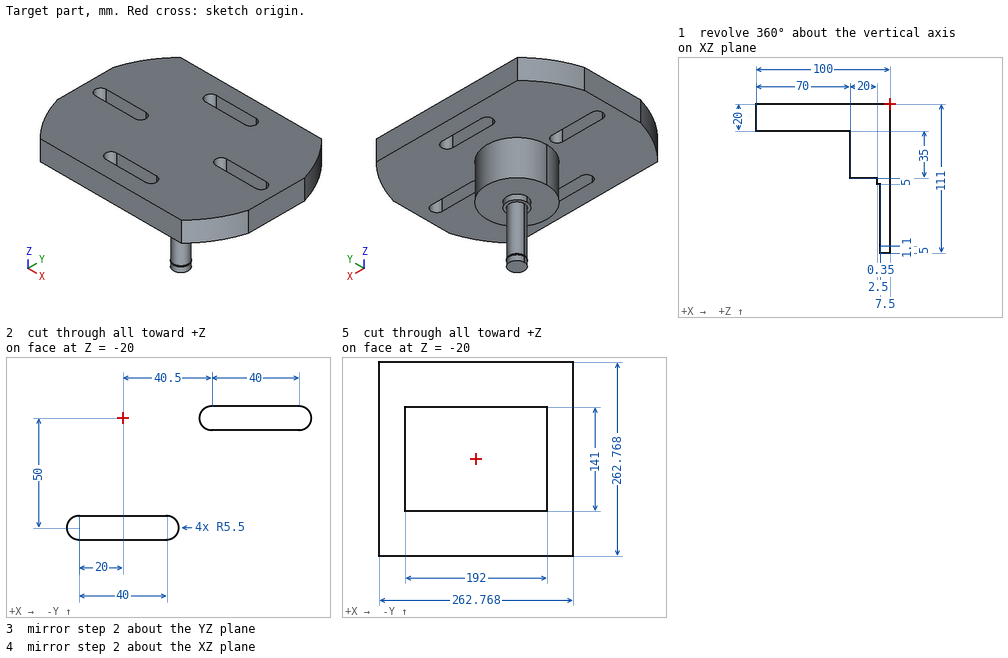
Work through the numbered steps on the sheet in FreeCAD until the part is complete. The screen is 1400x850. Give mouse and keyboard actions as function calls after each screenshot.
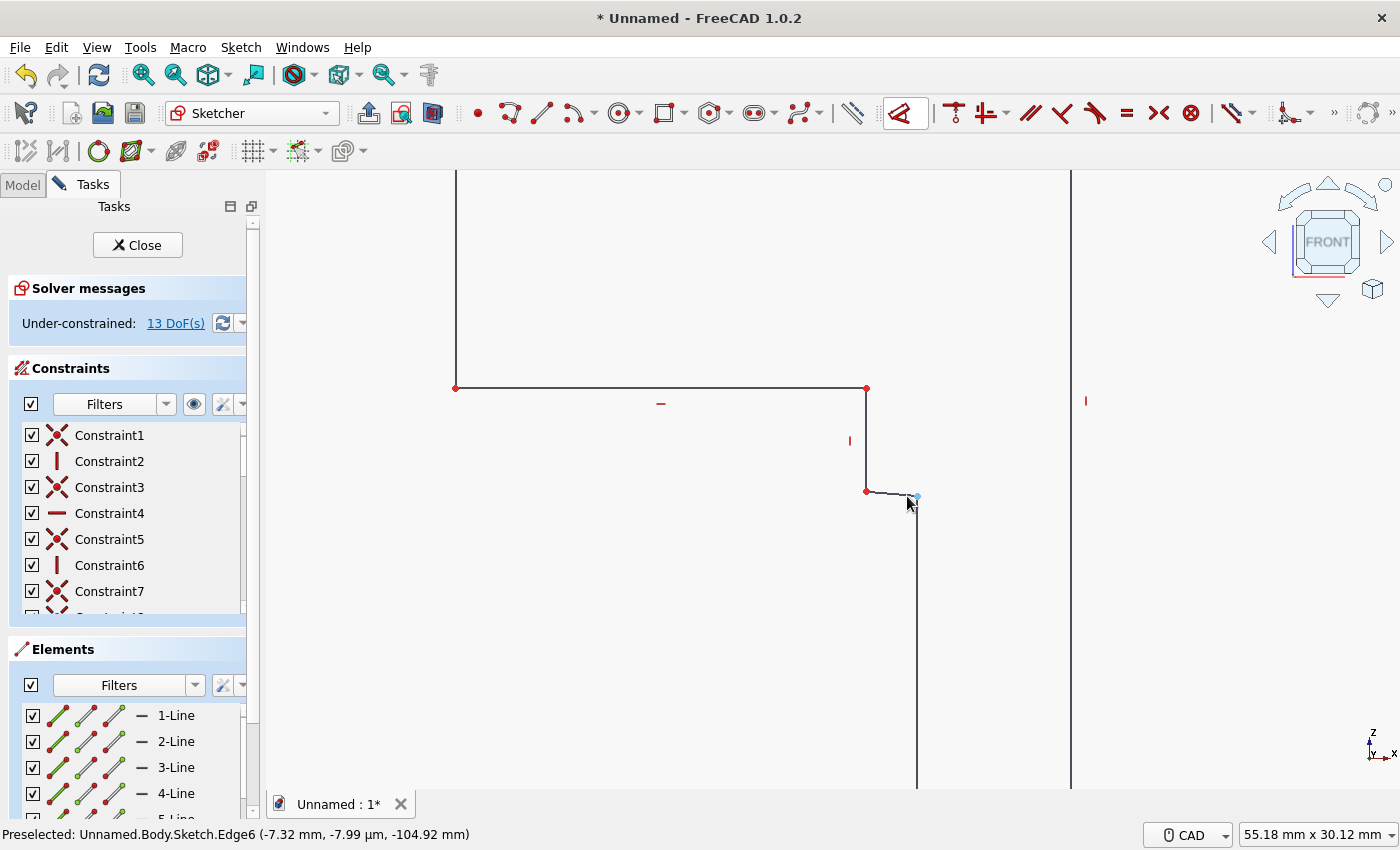
click(902, 495)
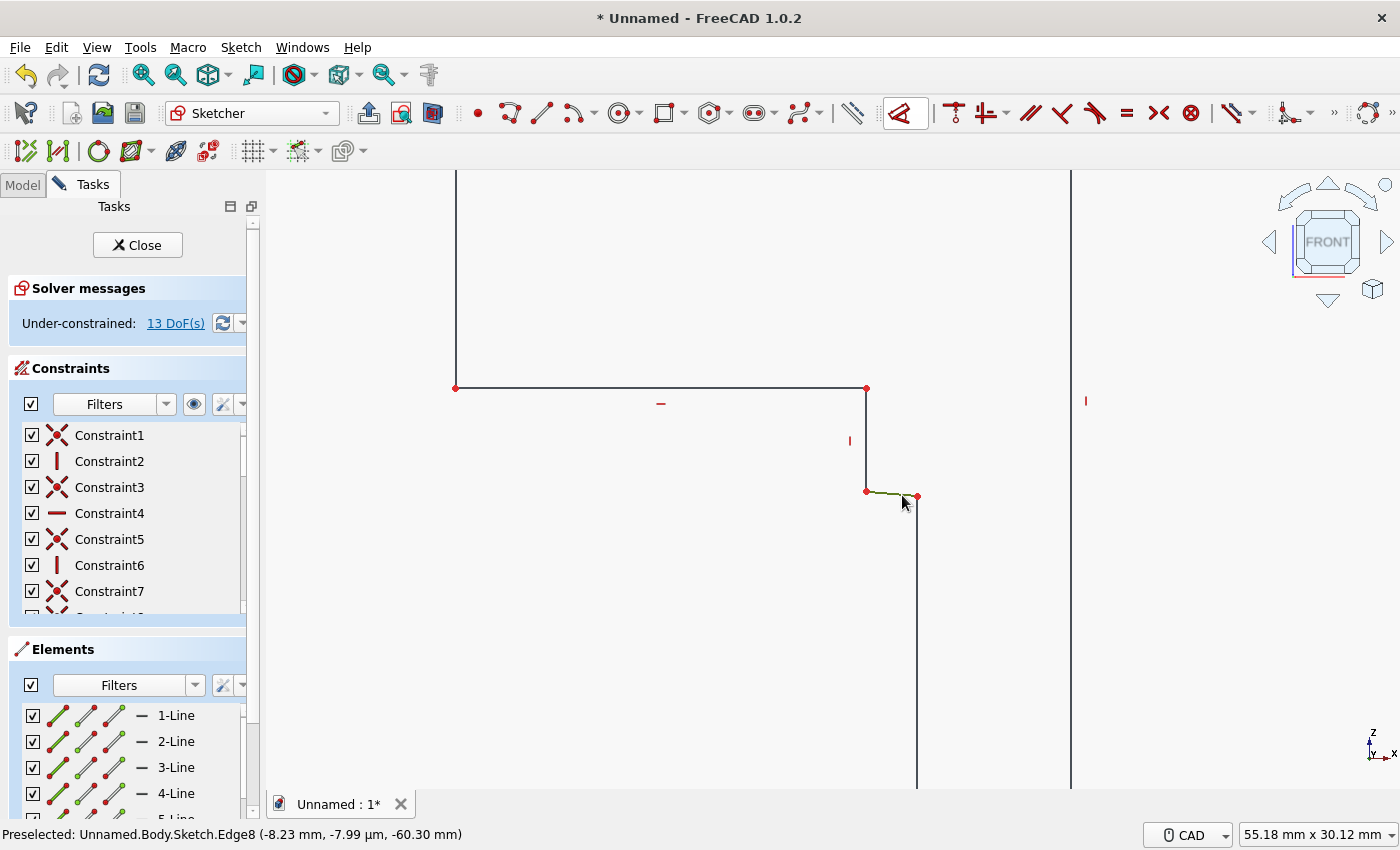
click(1008, 114)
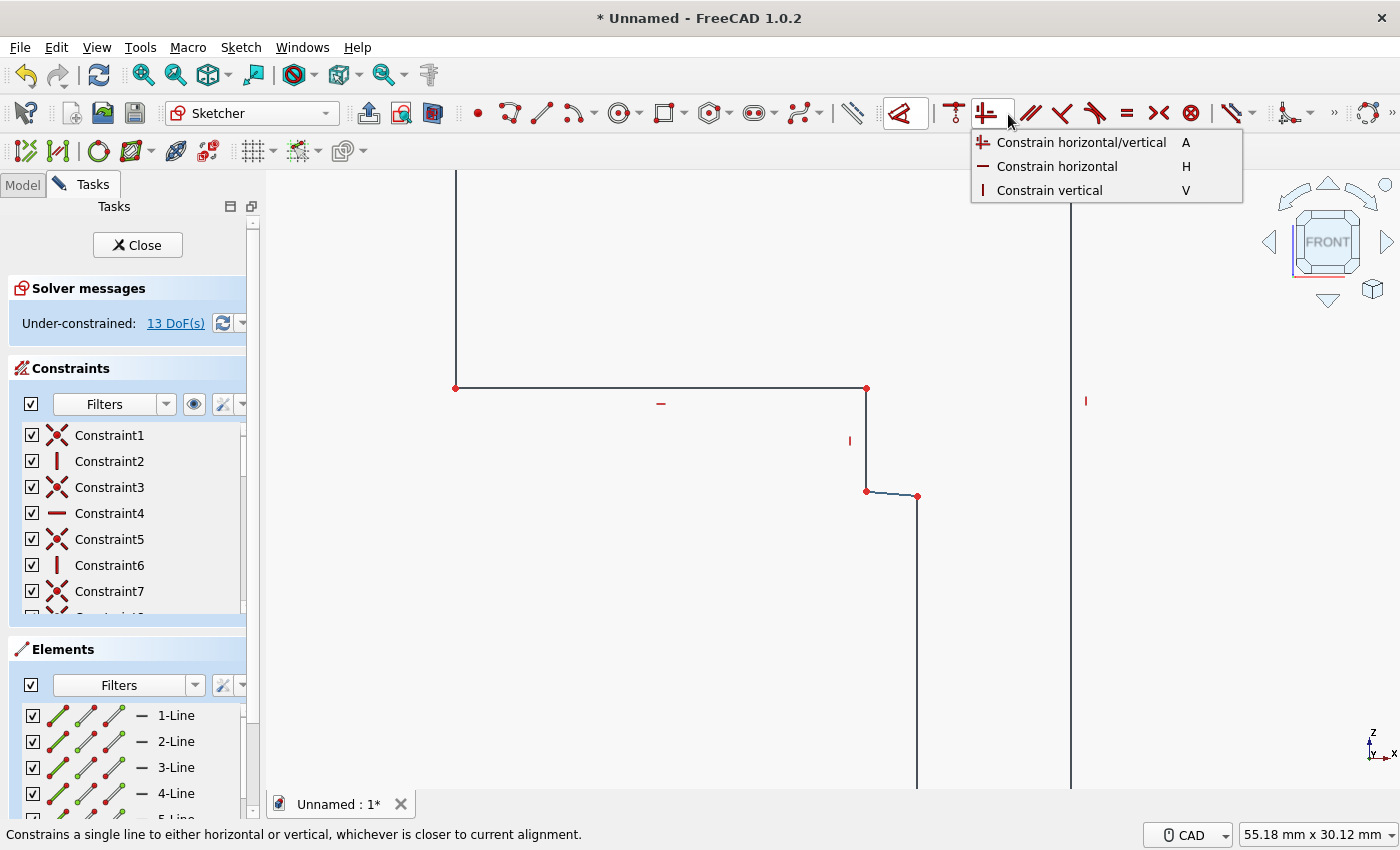
click(1107, 166)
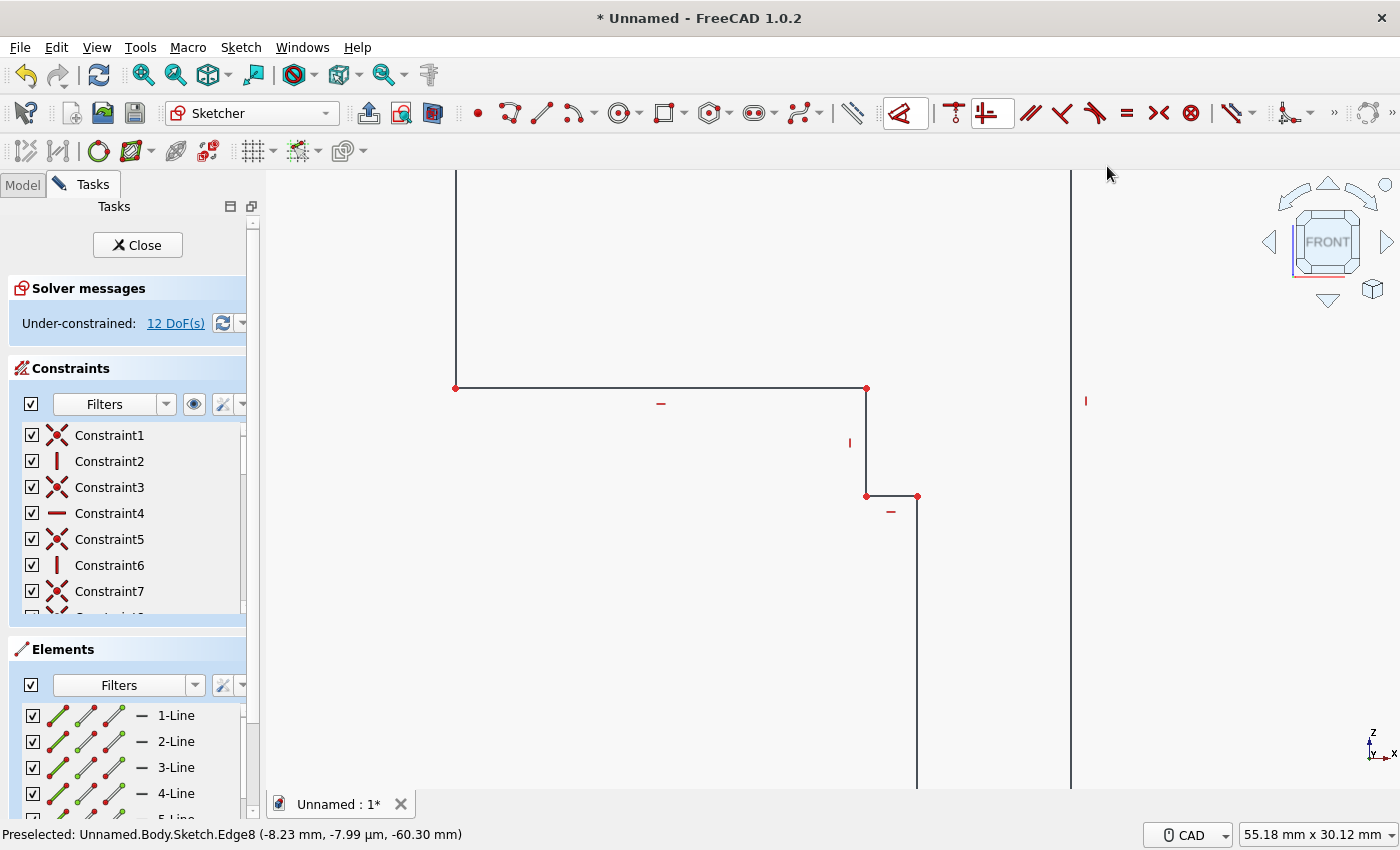
click(900, 114)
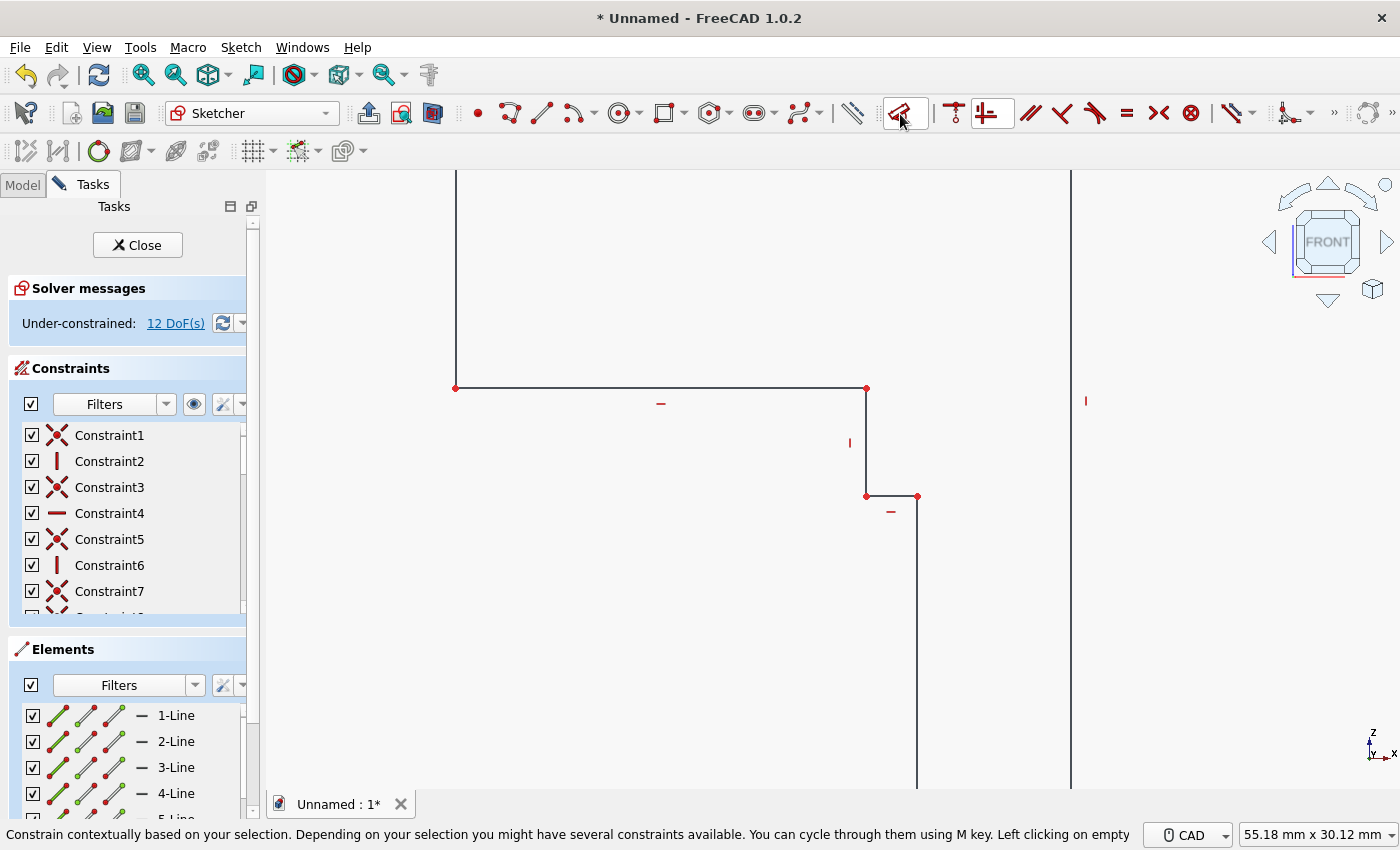
scroll(907, 496, down, 9)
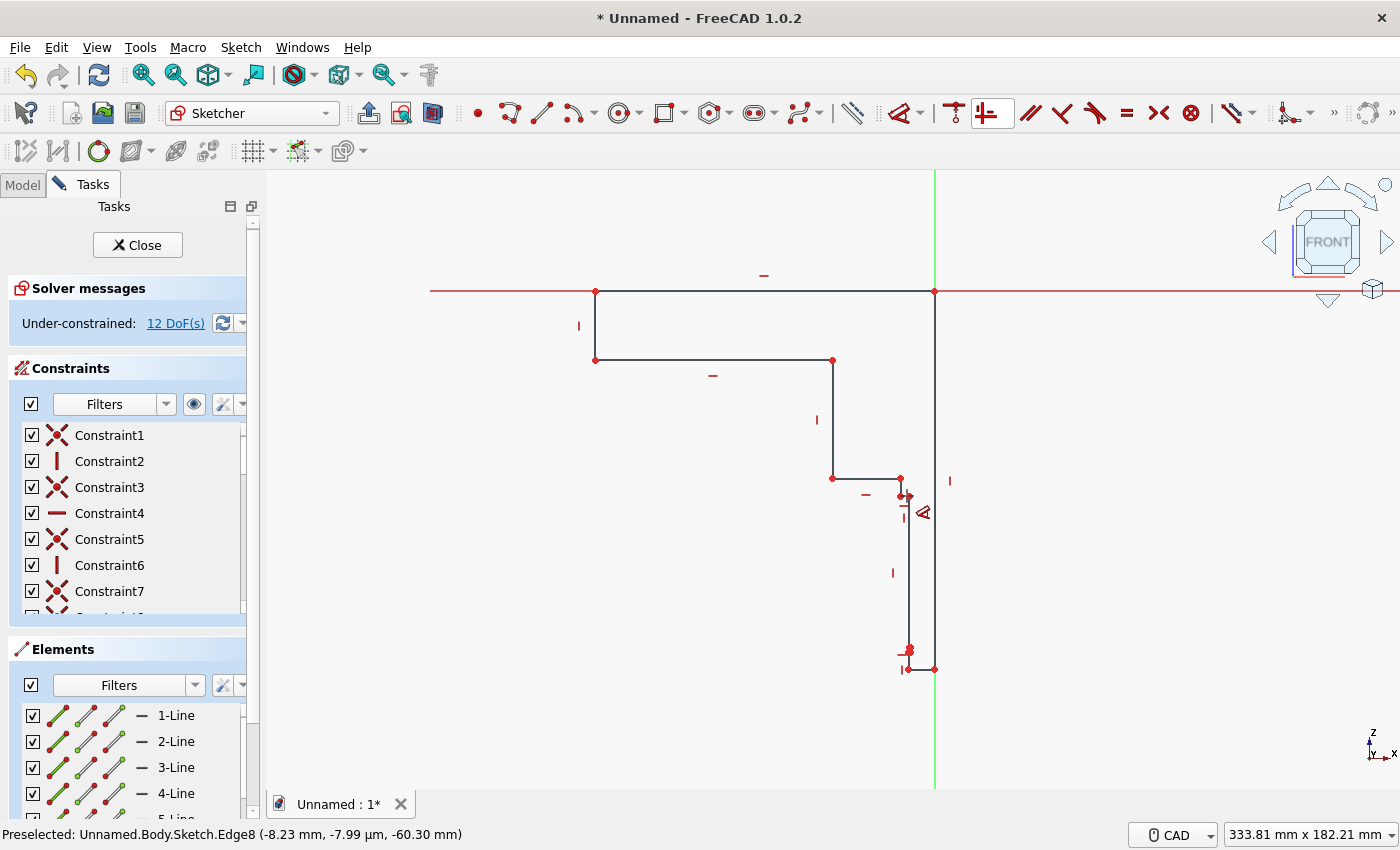
scroll(909, 665, up, 5)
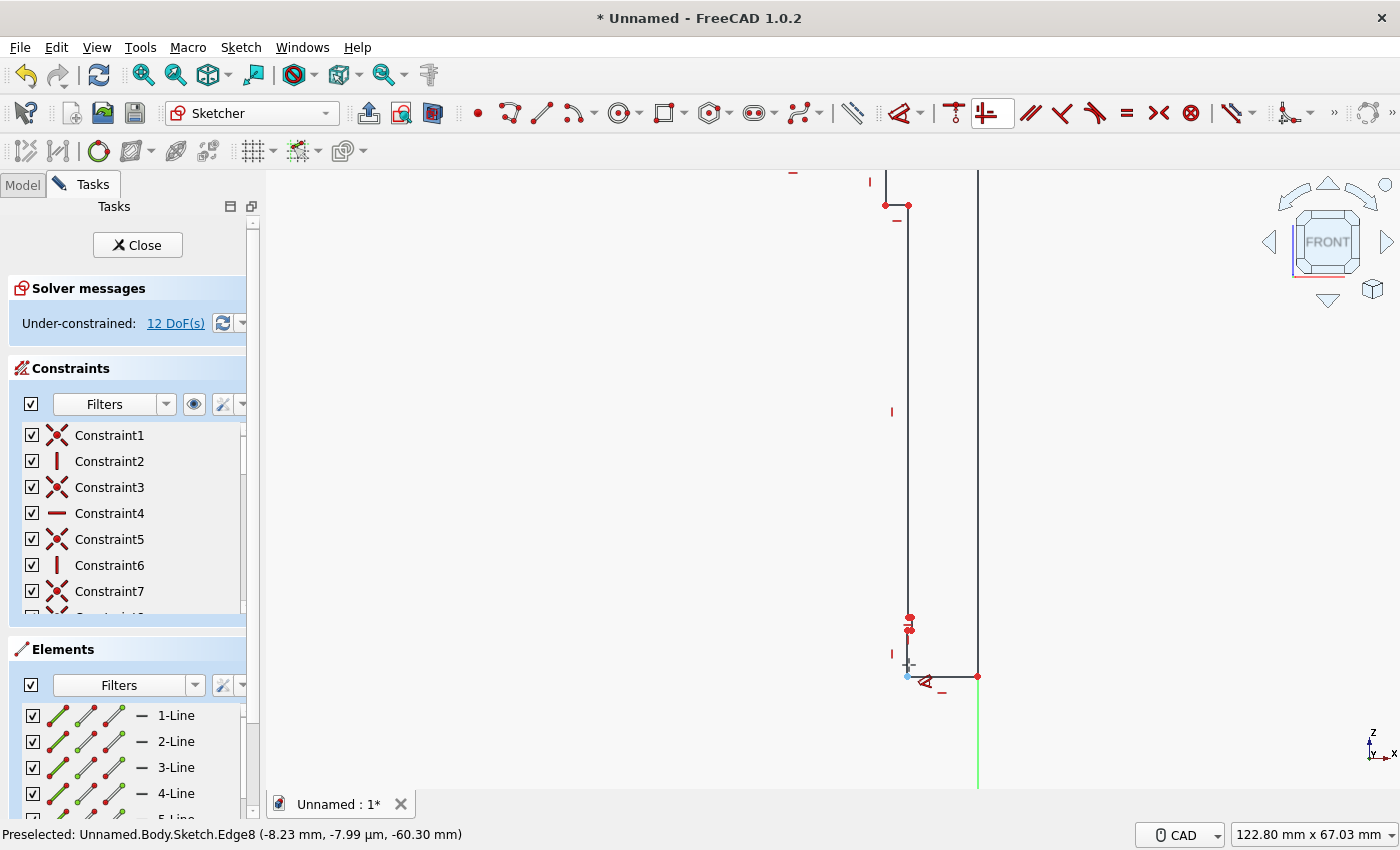
click(907, 663)
click(941, 654)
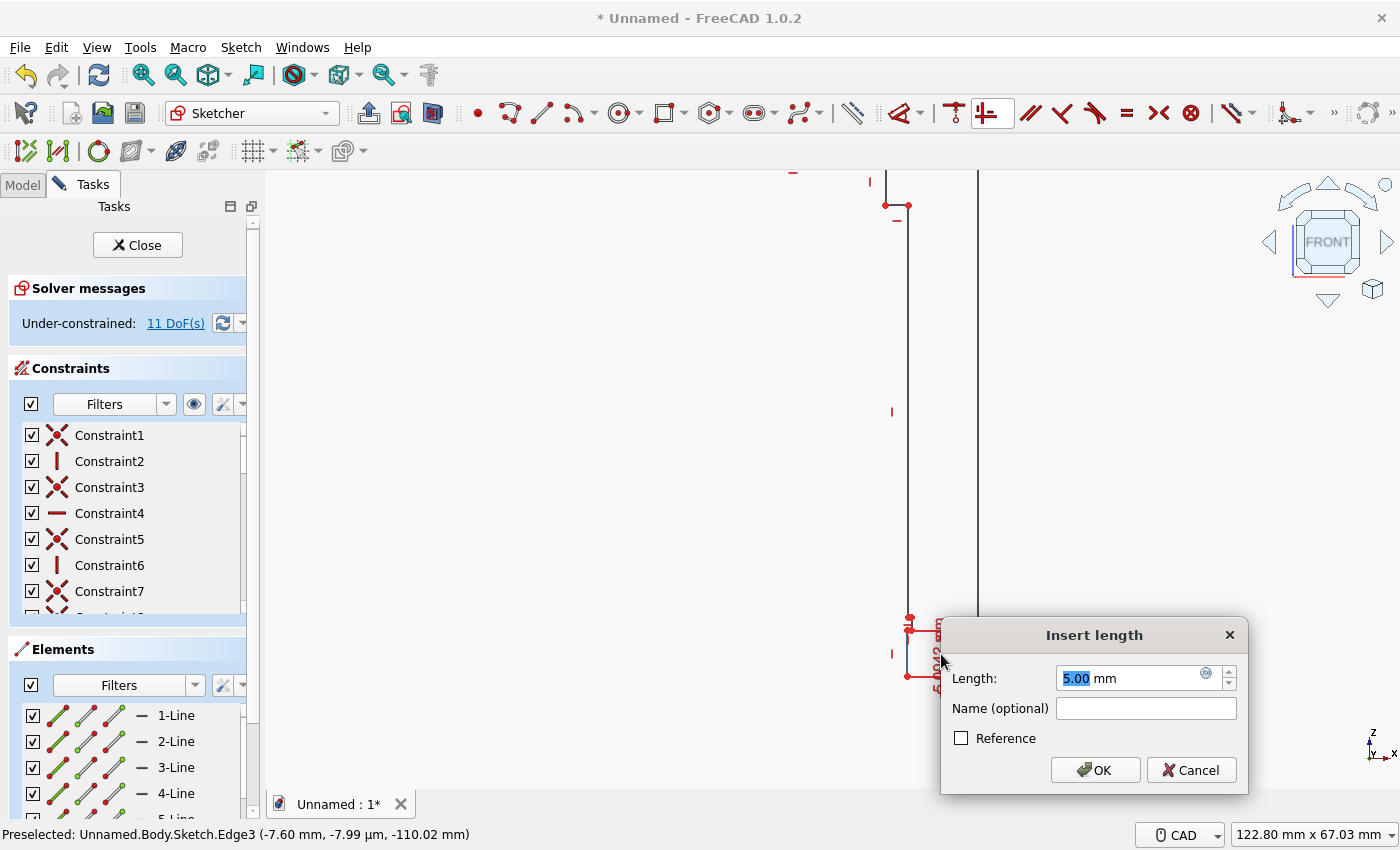
text(5)
key(Return)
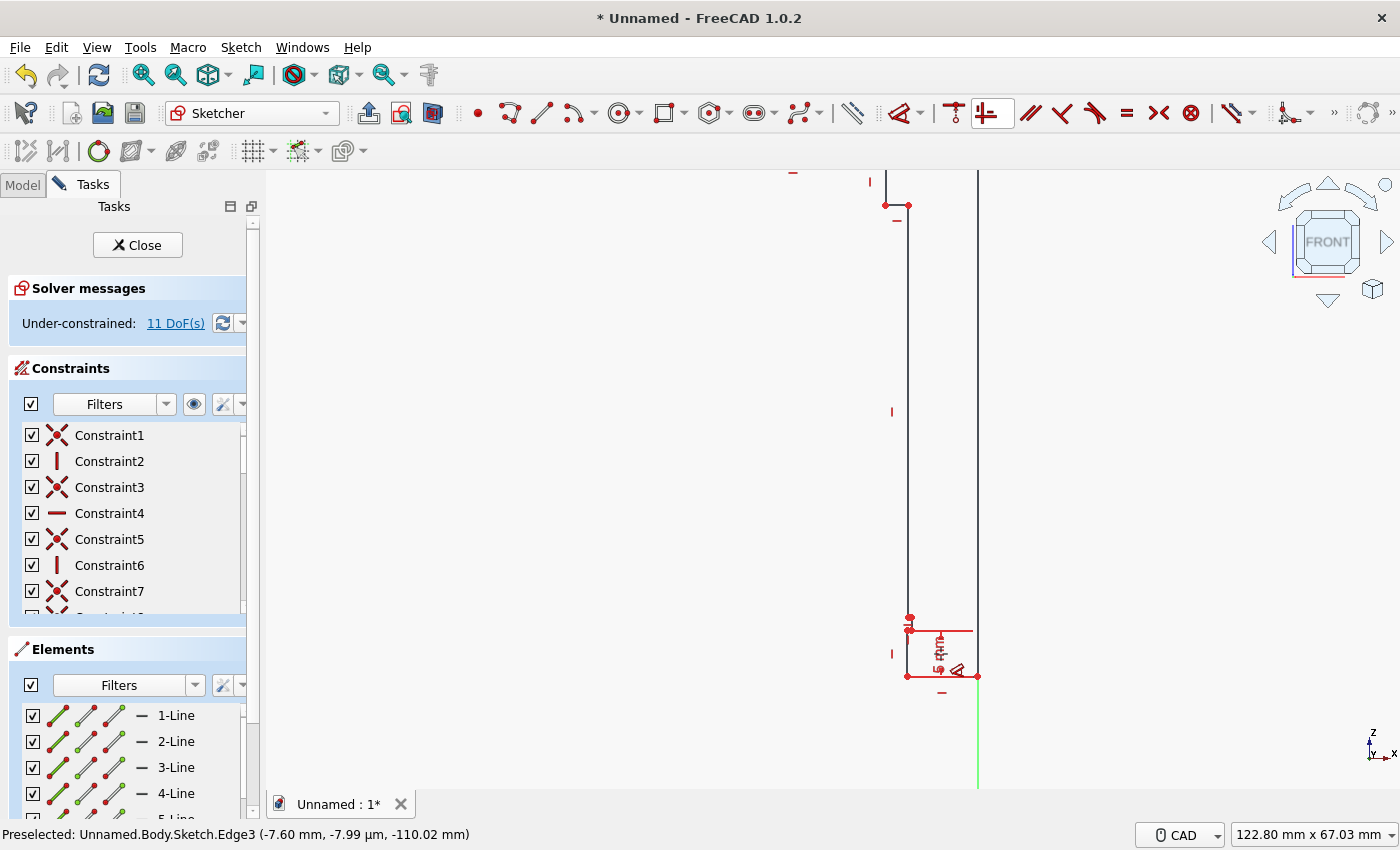
scroll(909, 665, down, 5)